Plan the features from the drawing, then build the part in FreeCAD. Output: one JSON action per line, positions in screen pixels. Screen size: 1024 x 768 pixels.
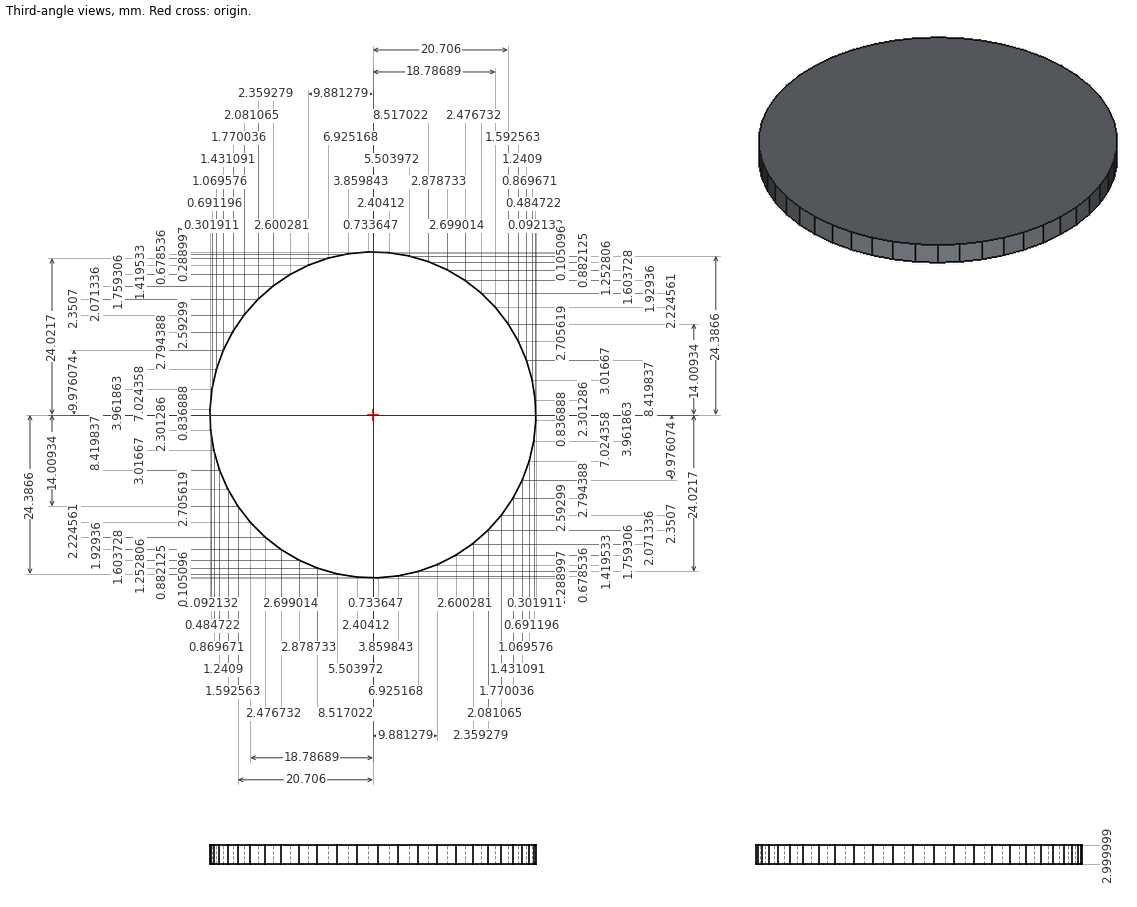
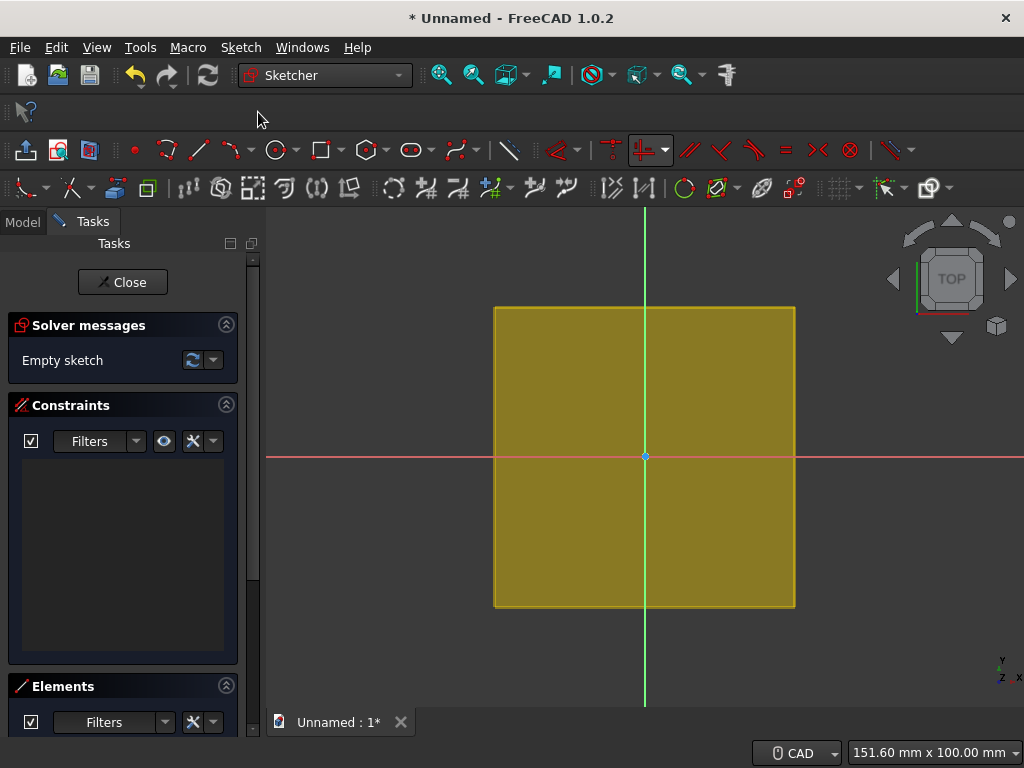
{"action": "left_click", "coordinate": [168, 150]}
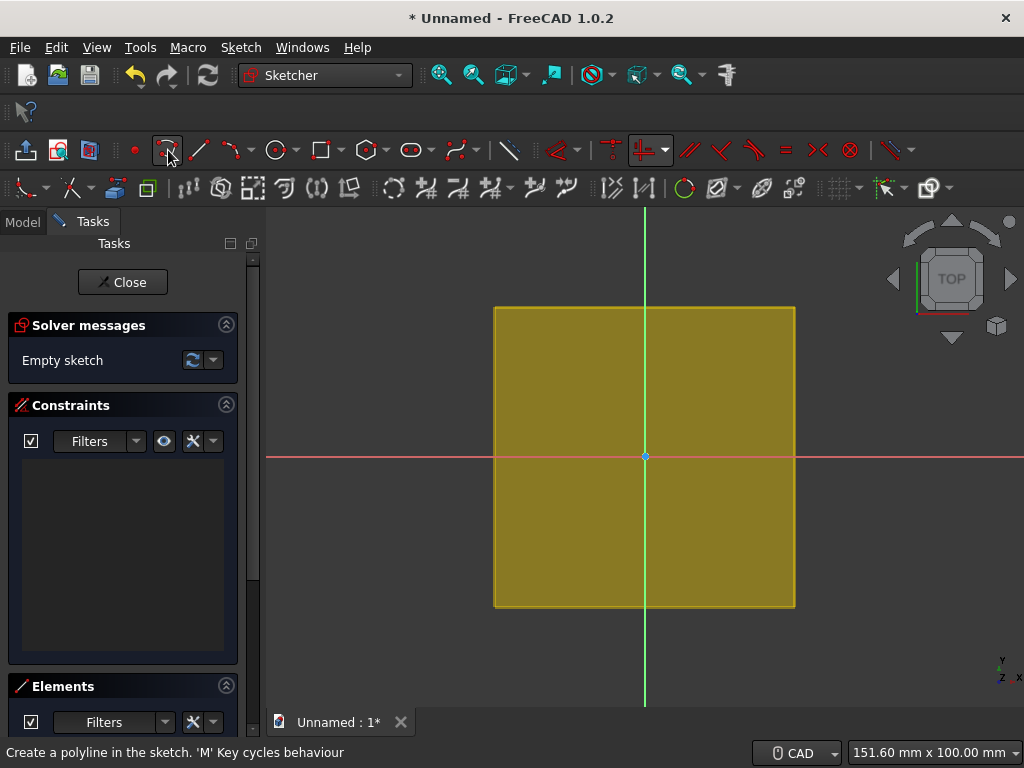
{"action": "left_click", "coordinate": [673, 335]}
{"action": "left_click", "coordinate": [688, 339]}
{"action": "left_click", "coordinate": [702, 346]}
{"action": "left_click", "coordinate": [715, 354]}
{"action": "left_click", "coordinate": [728, 363]}
{"action": "left_click", "coordinate": [739, 375]}
{"action": "left_click", "coordinate": [749, 387]}
{"action": "left_click", "coordinate": [756, 400]}
{"action": "left_click", "coordinate": [763, 415]}
{"action": "left_click", "coordinate": [767, 430]}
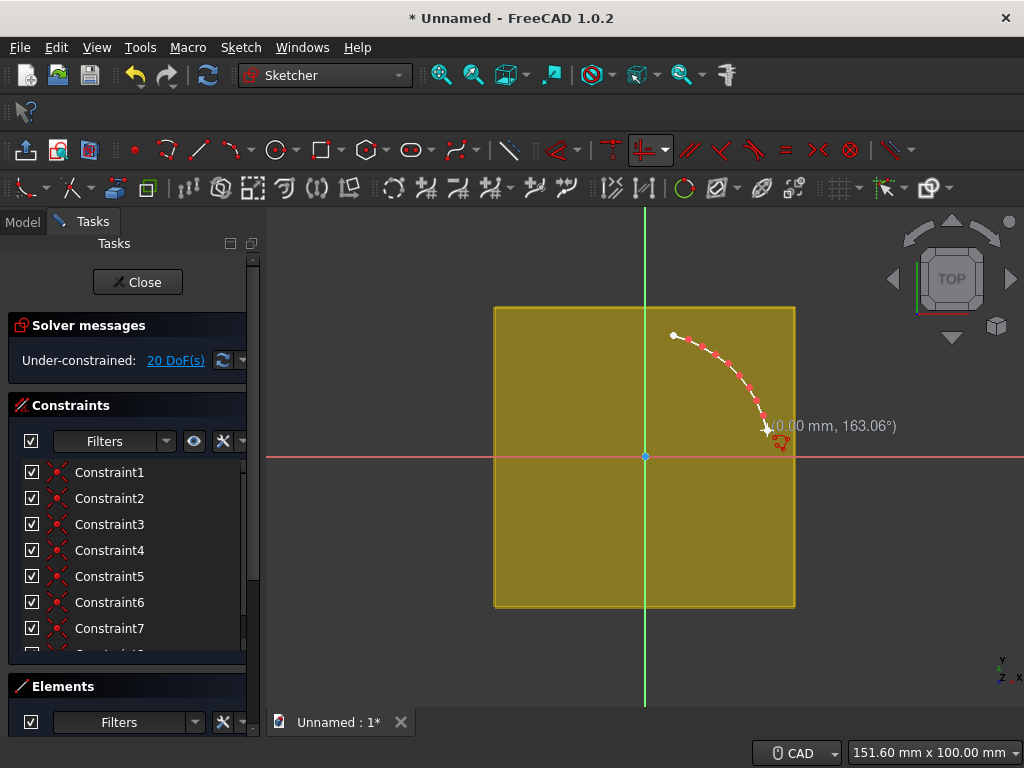
{"action": "scroll", "coordinate": [769, 445], "scroll_direction": "up", "scroll_amount": 2}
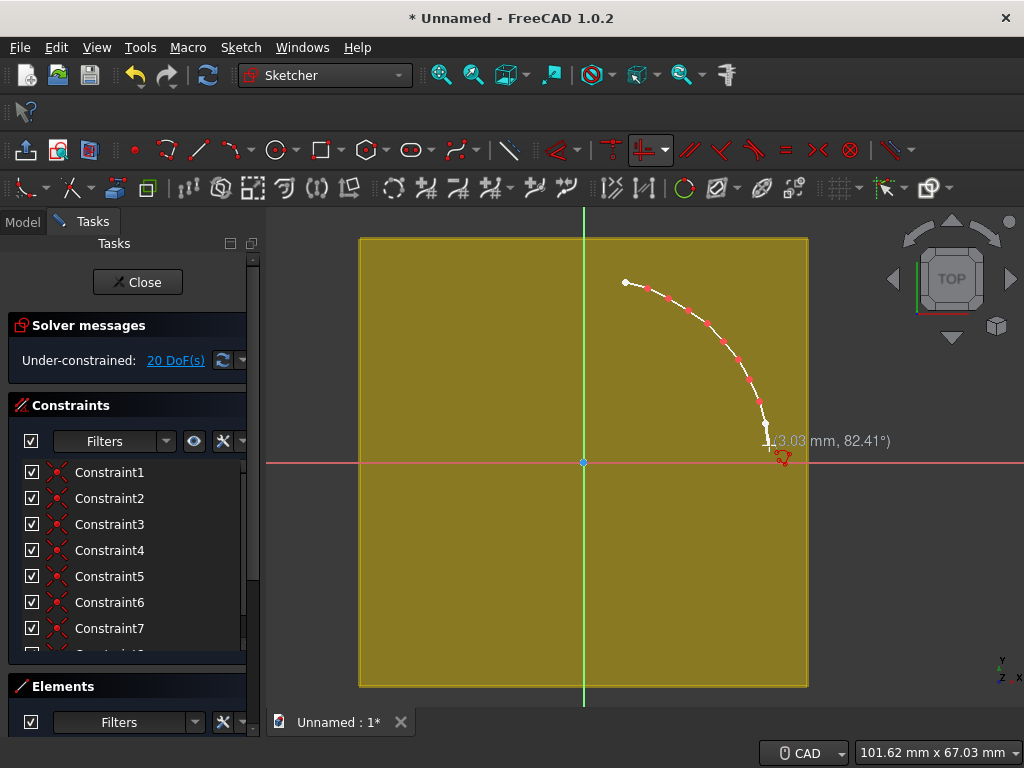
{"action": "left_click", "coordinate": [769, 446]}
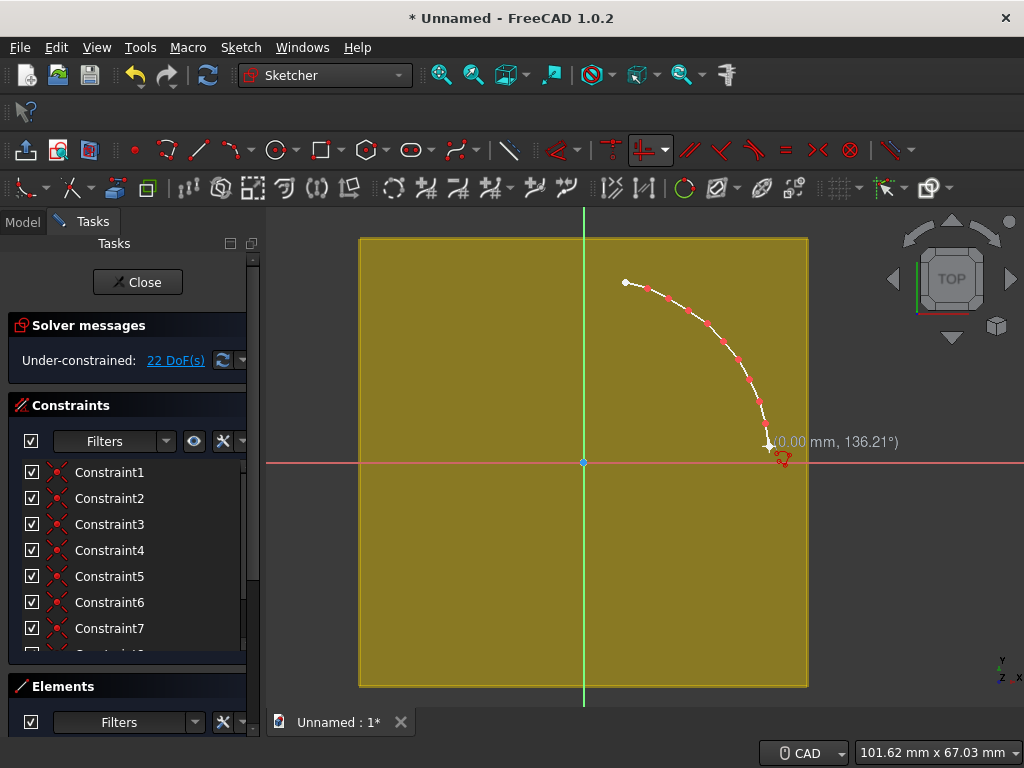
{"action": "scroll", "coordinate": [770, 469], "scroll_direction": "up", "scroll_amount": 5}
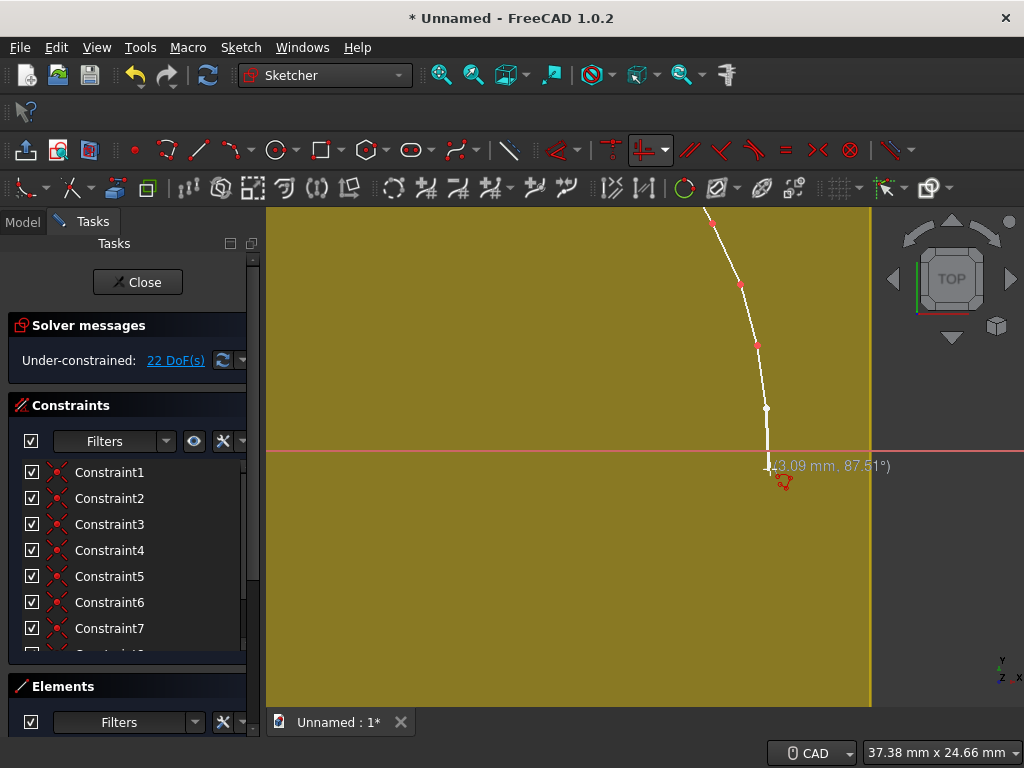
{"action": "left_click", "coordinate": [771, 468]}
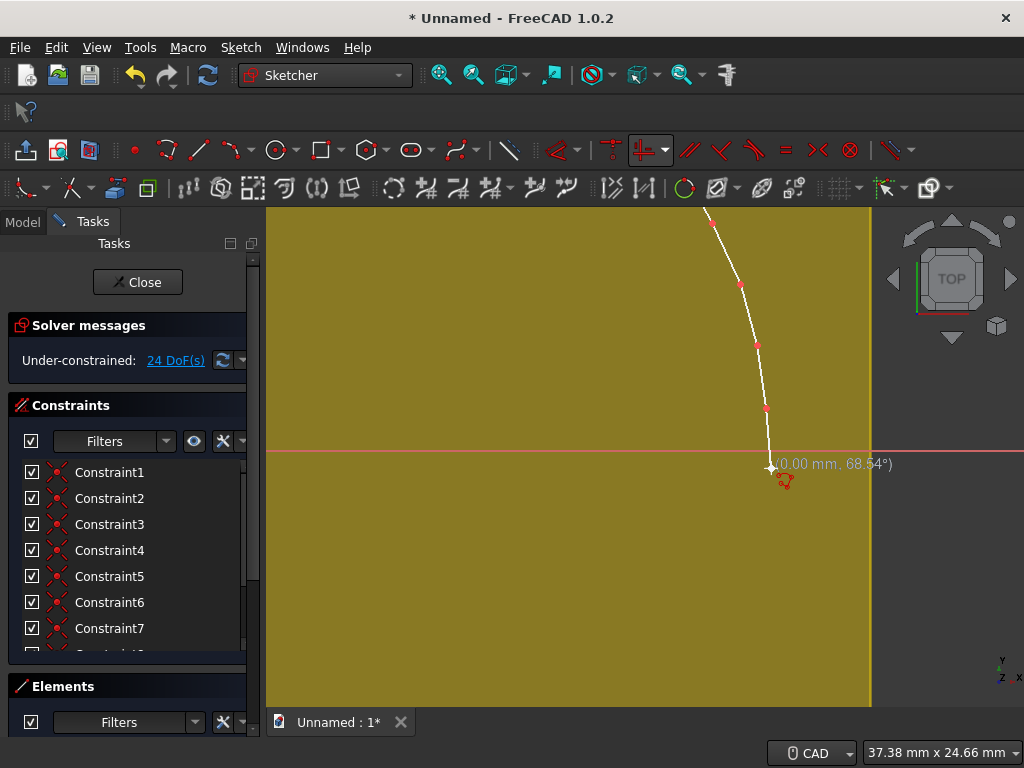
{"action": "scroll", "coordinate": [712, 460], "scroll_direction": "down", "scroll_amount": 6}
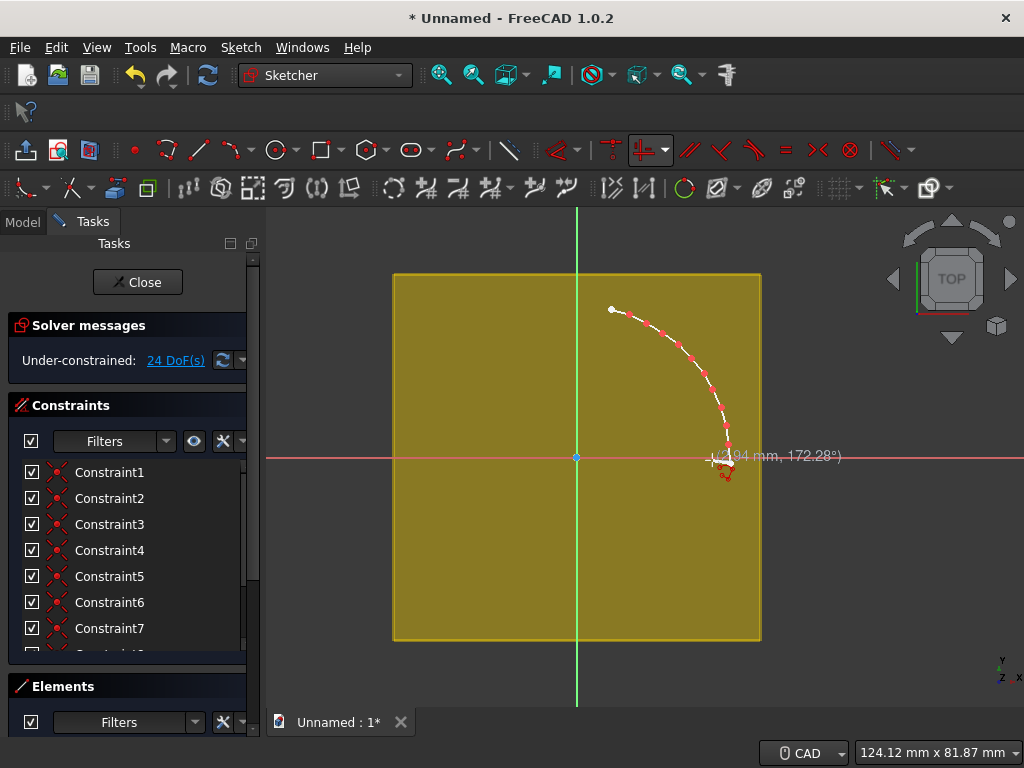
{"action": "left_click", "coordinate": [728, 482]}
{"action": "left_click", "coordinate": [724, 501]}
{"action": "left_click", "coordinate": [717, 519]}
{"action": "left_click", "coordinate": [708, 536]}
{"action": "left_click", "coordinate": [697, 551]}
{"action": "left_click", "coordinate": [685, 566]}
{"action": "left_click", "coordinate": [670, 578]}
{"action": "left_click", "coordinate": [654, 589]}
{"action": "left_click", "coordinate": [637, 598]}
{"action": "left_click", "coordinate": [619, 604]}
{"action": "left_click", "coordinate": [601, 608]}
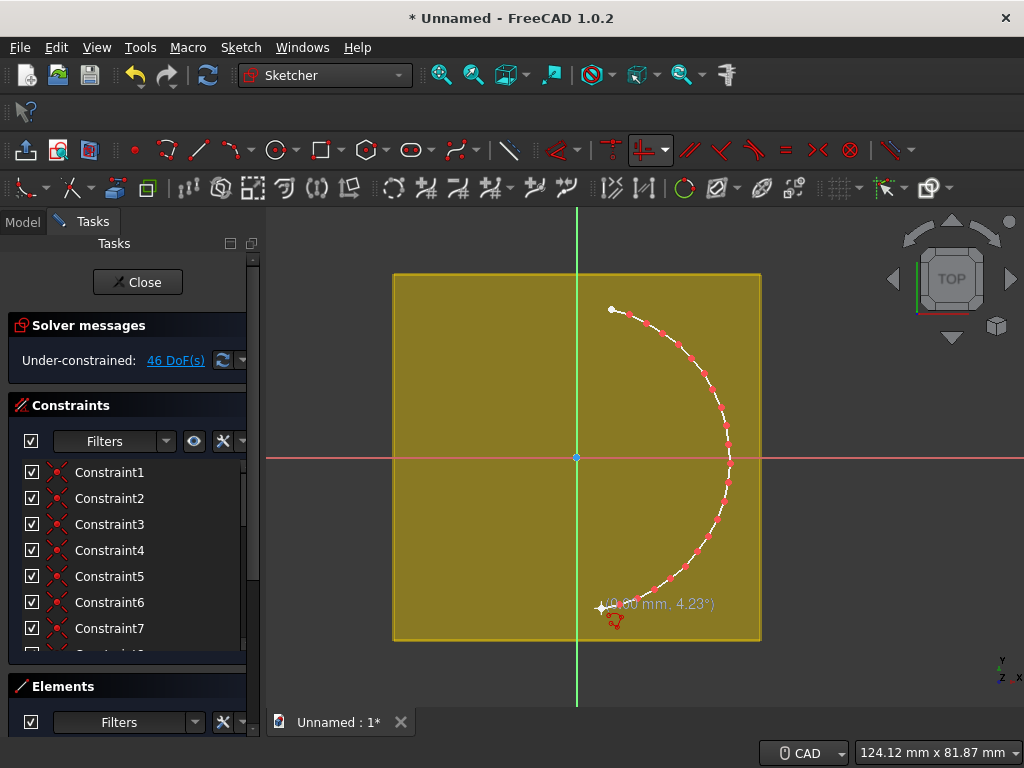
{"action": "scroll", "coordinate": [581, 610], "scroll_direction": "up", "scroll_amount": 7}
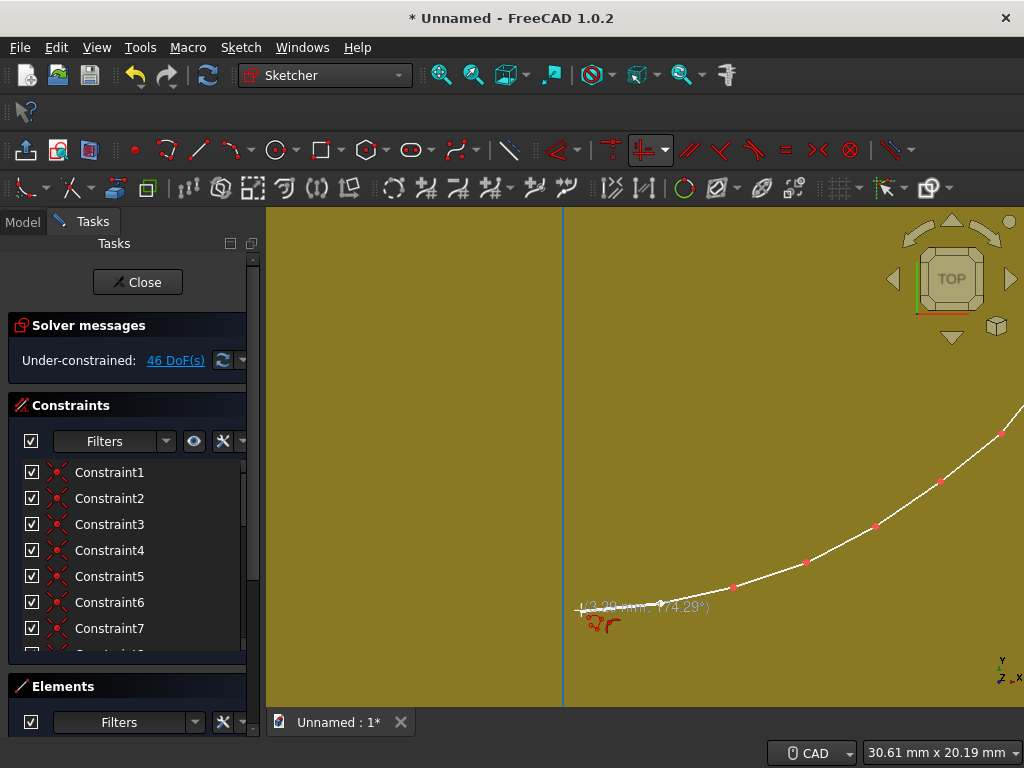
{"action": "left_click", "coordinate": [582, 608]}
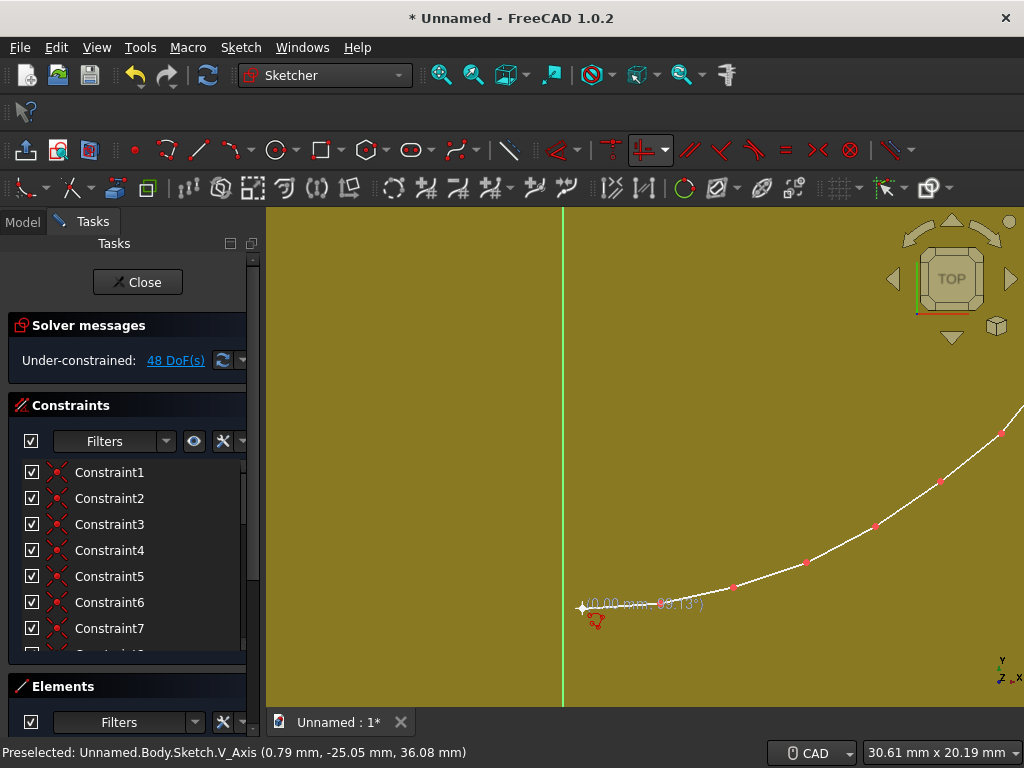
{"action": "scroll", "coordinate": [581, 610], "scroll_direction": "down", "scroll_amount": 7}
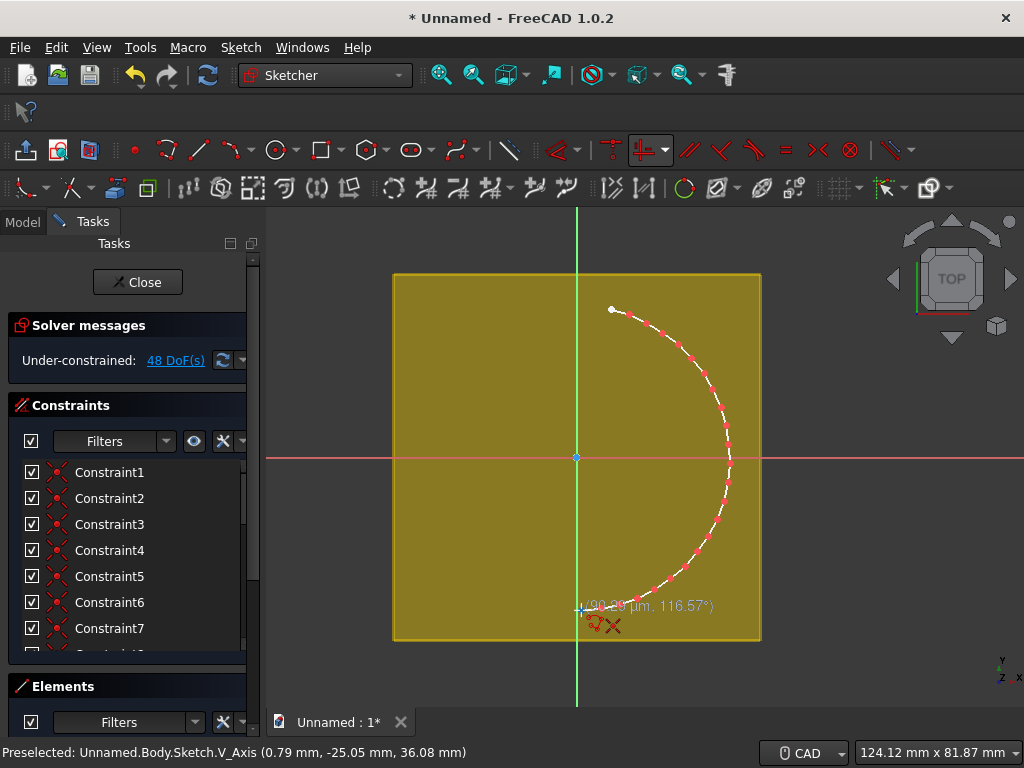
{"action": "left_click", "coordinate": [562, 608]}
{"action": "left_click", "coordinate": [543, 607]}
{"action": "left_click", "coordinate": [525, 601]}
{"action": "left_click", "coordinate": [507, 593]}
{"action": "left_click", "coordinate": [491, 584]}
{"action": "left_click", "coordinate": [476, 572]}
{"action": "left_click", "coordinate": [462, 558]}
{"action": "left_click", "coordinate": [451, 543]}
{"action": "left_click", "coordinate": [441, 527]}
{"action": "left_click", "coordinate": [433, 509]}
{"action": "left_click", "coordinate": [428, 491]}
{"action": "left_click", "coordinate": [425, 472]}